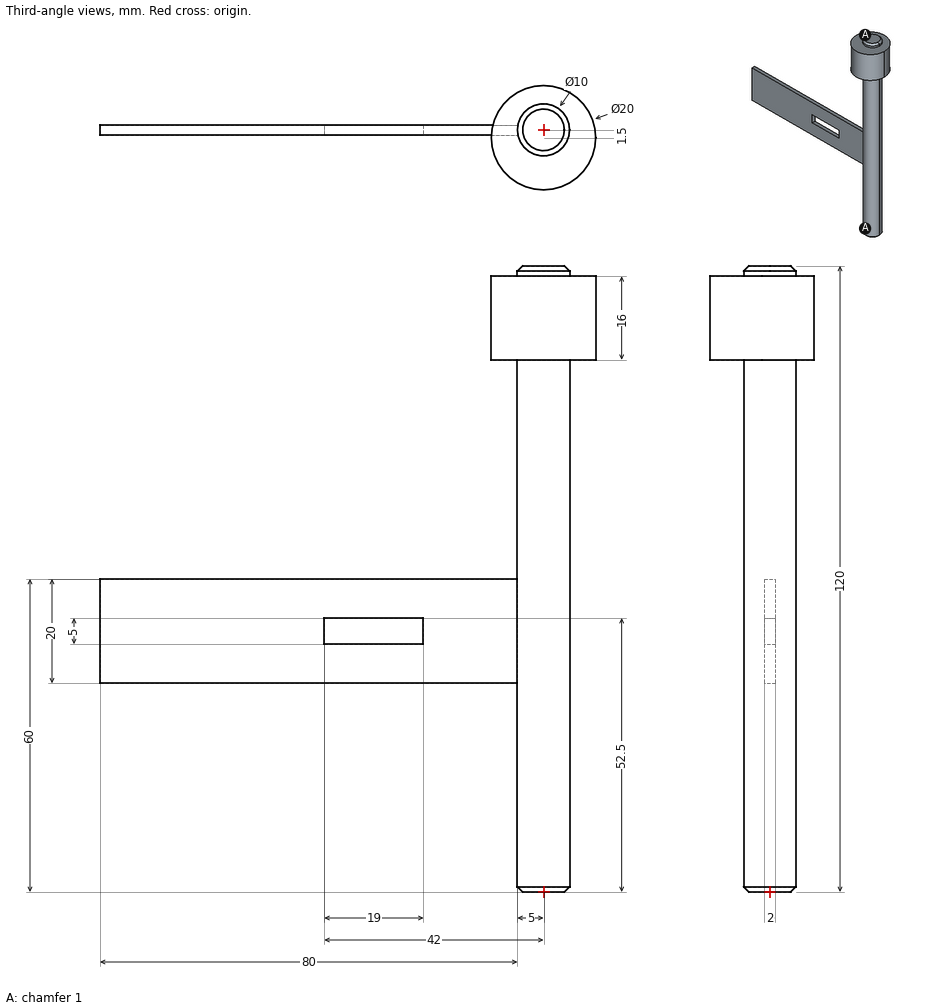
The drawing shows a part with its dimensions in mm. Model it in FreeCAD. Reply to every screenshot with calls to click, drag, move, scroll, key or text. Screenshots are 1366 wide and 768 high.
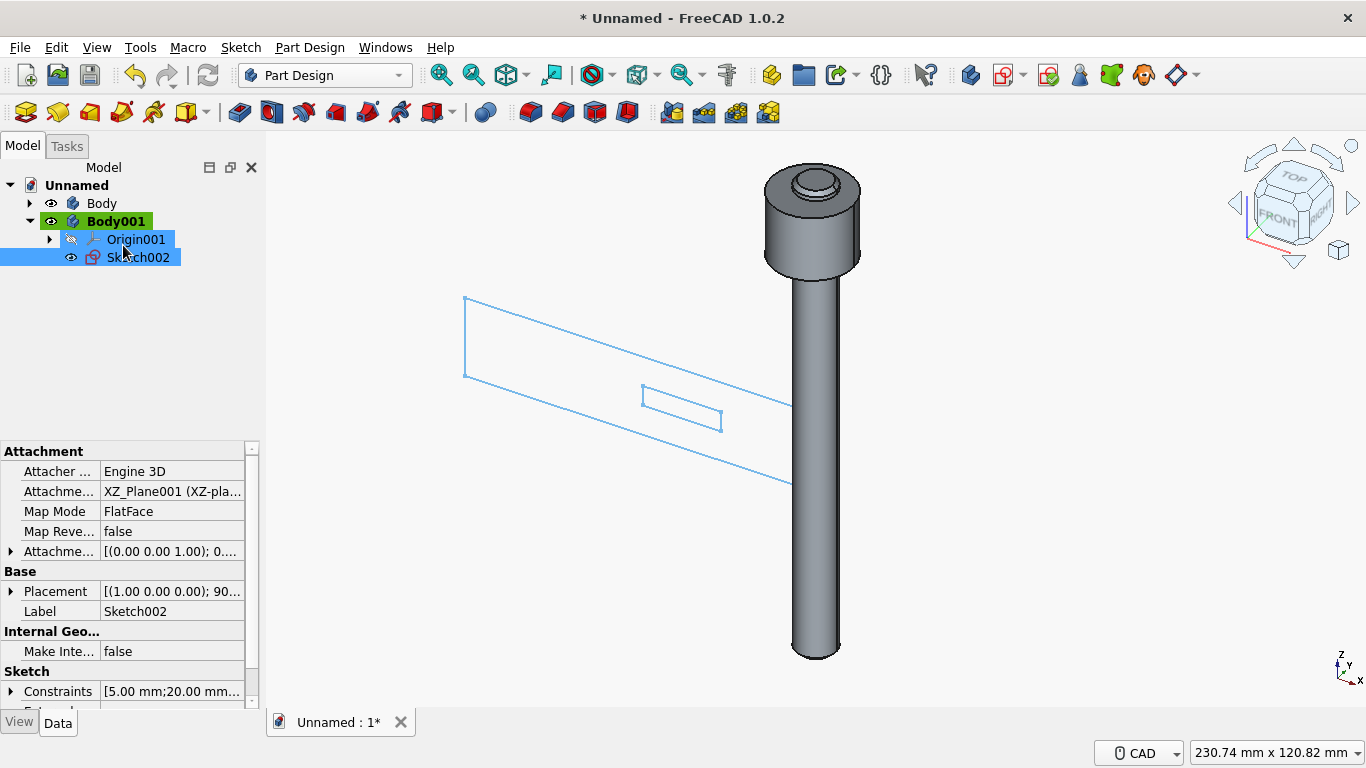
click(26, 112)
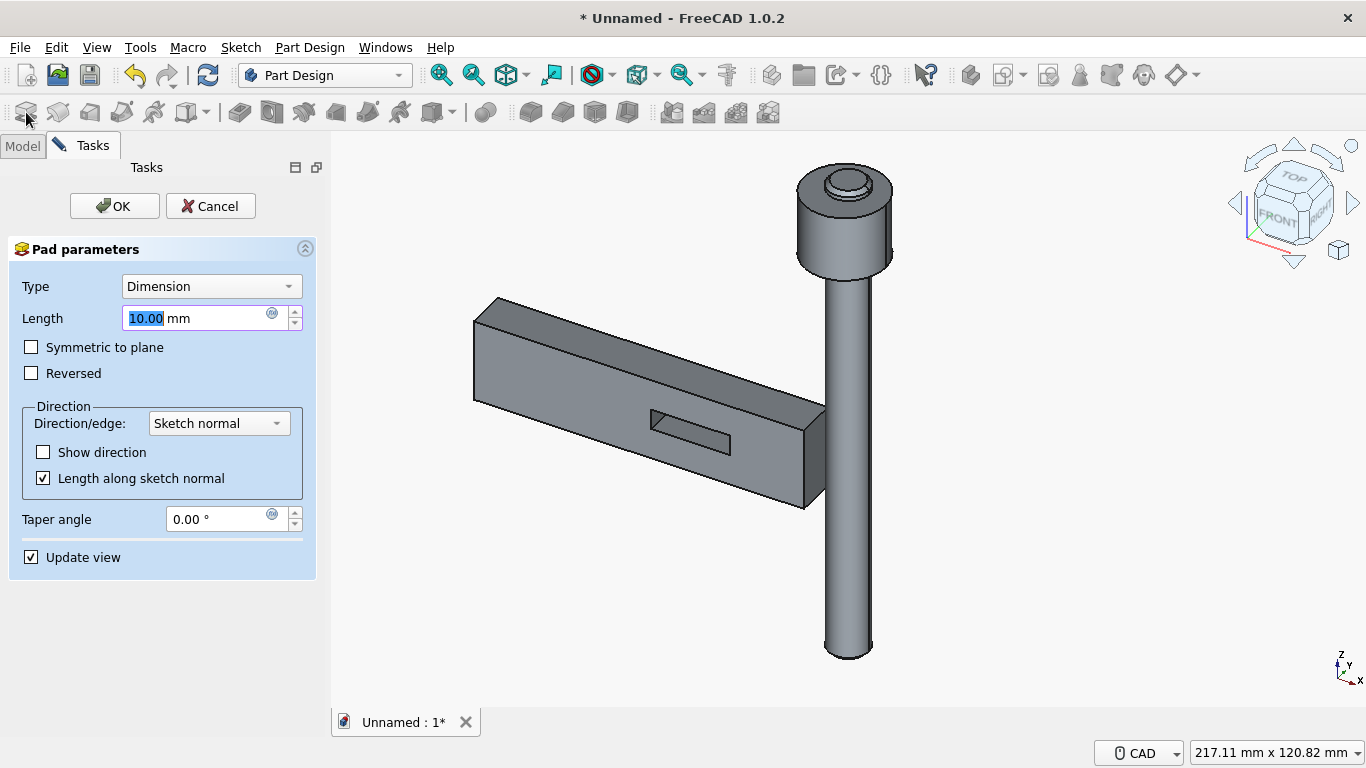
text(2)
key(Tab)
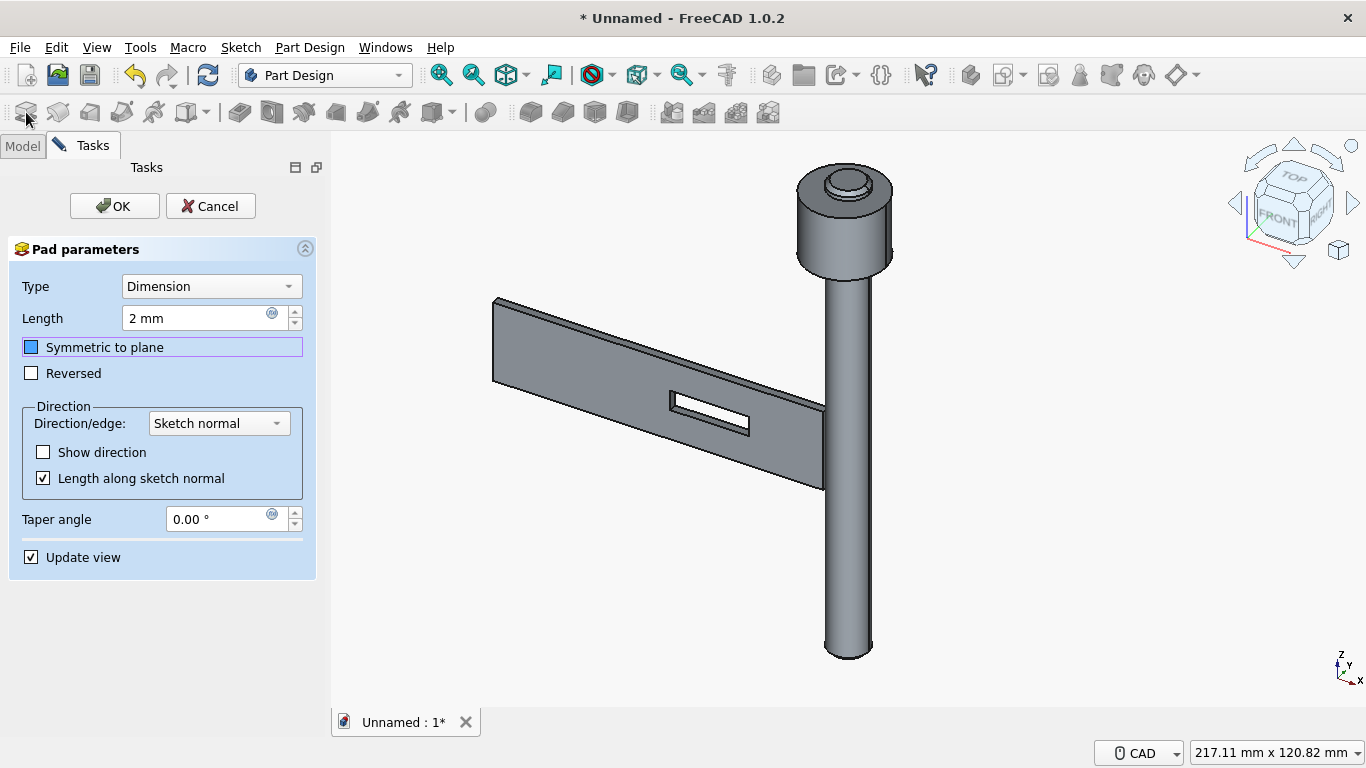
click(30, 347)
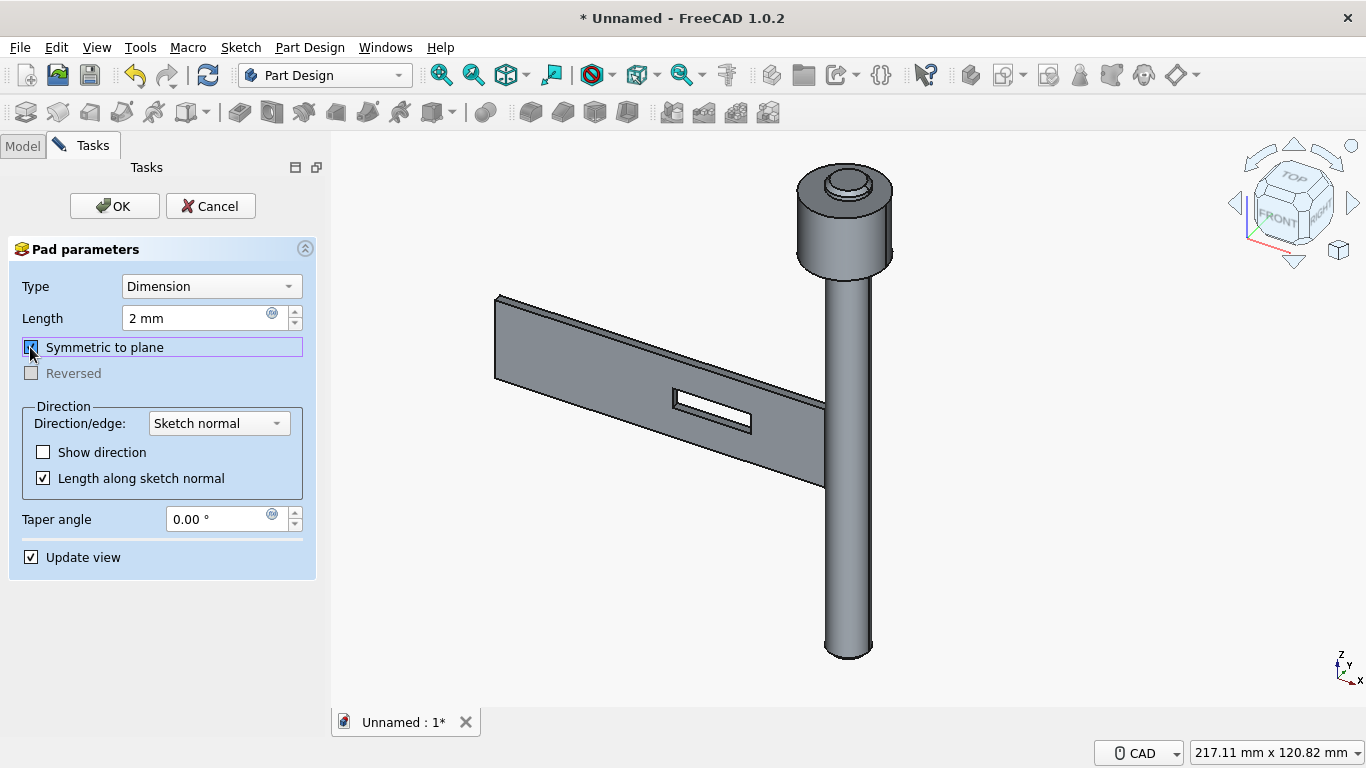
click(115, 206)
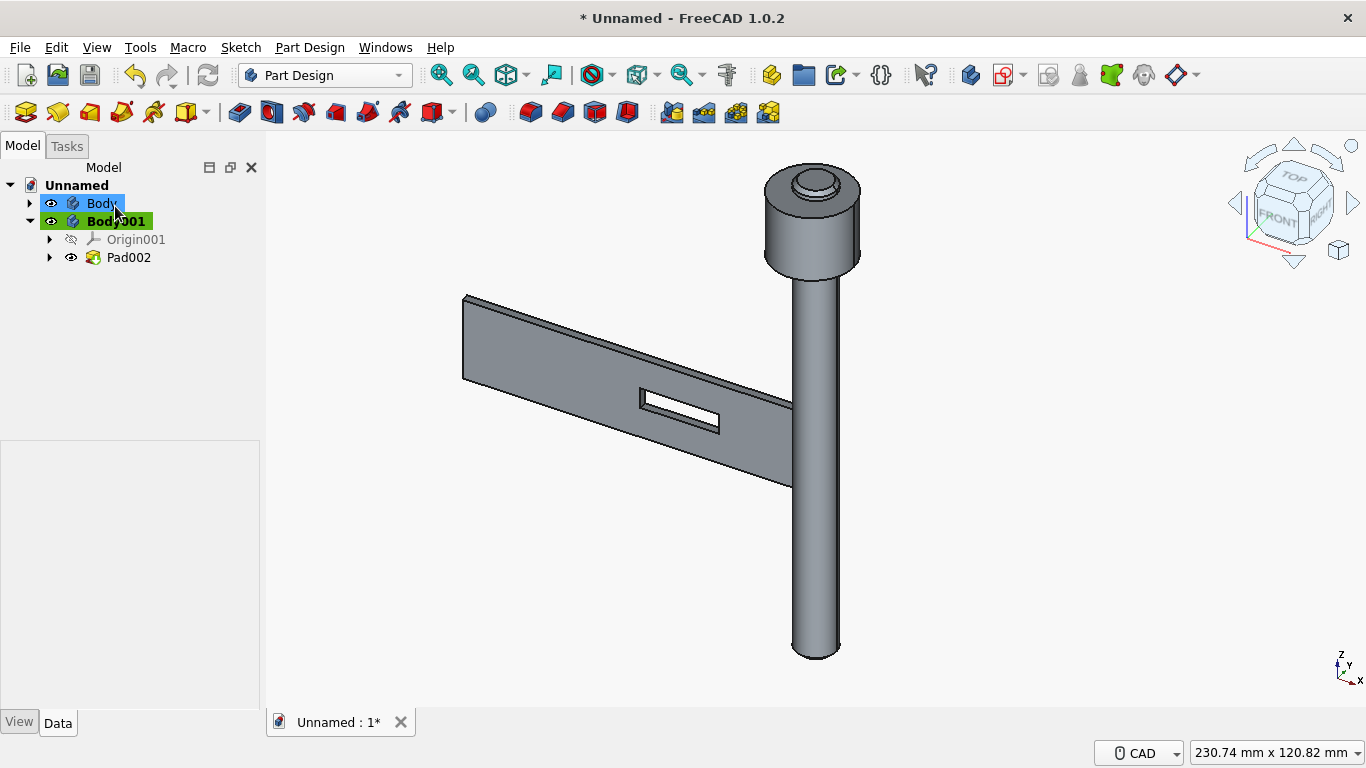
key(0)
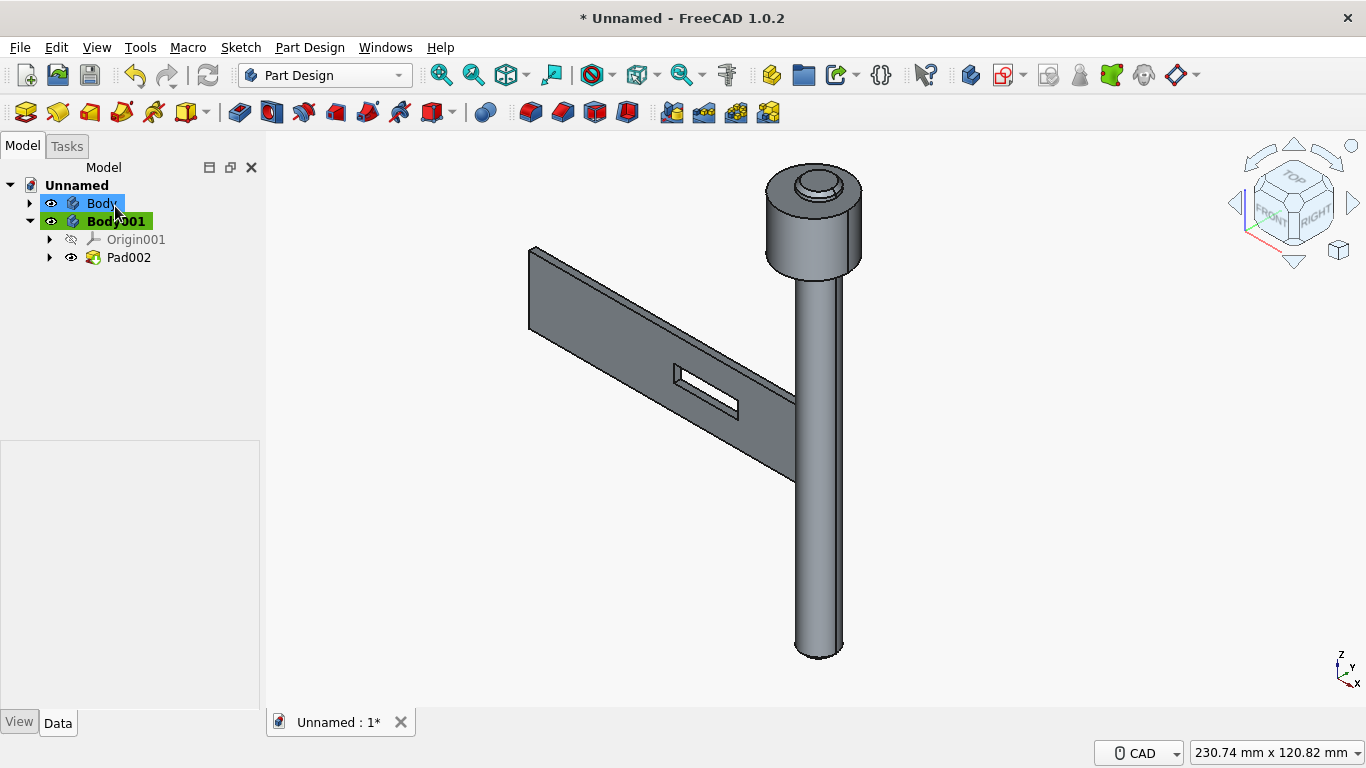
click(442, 76)